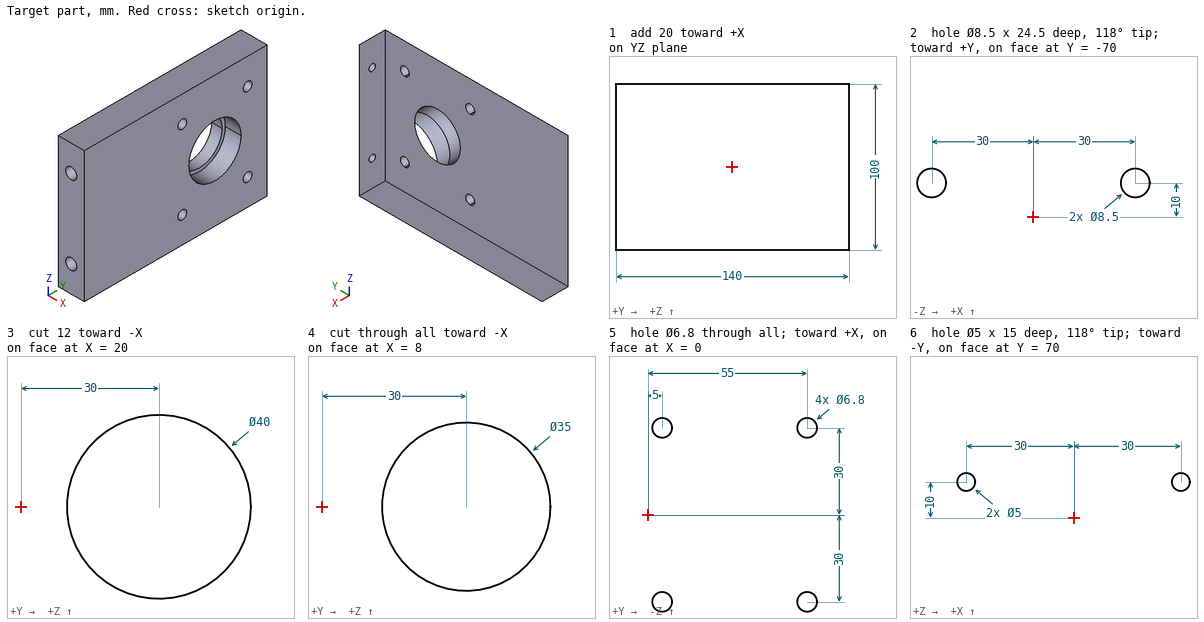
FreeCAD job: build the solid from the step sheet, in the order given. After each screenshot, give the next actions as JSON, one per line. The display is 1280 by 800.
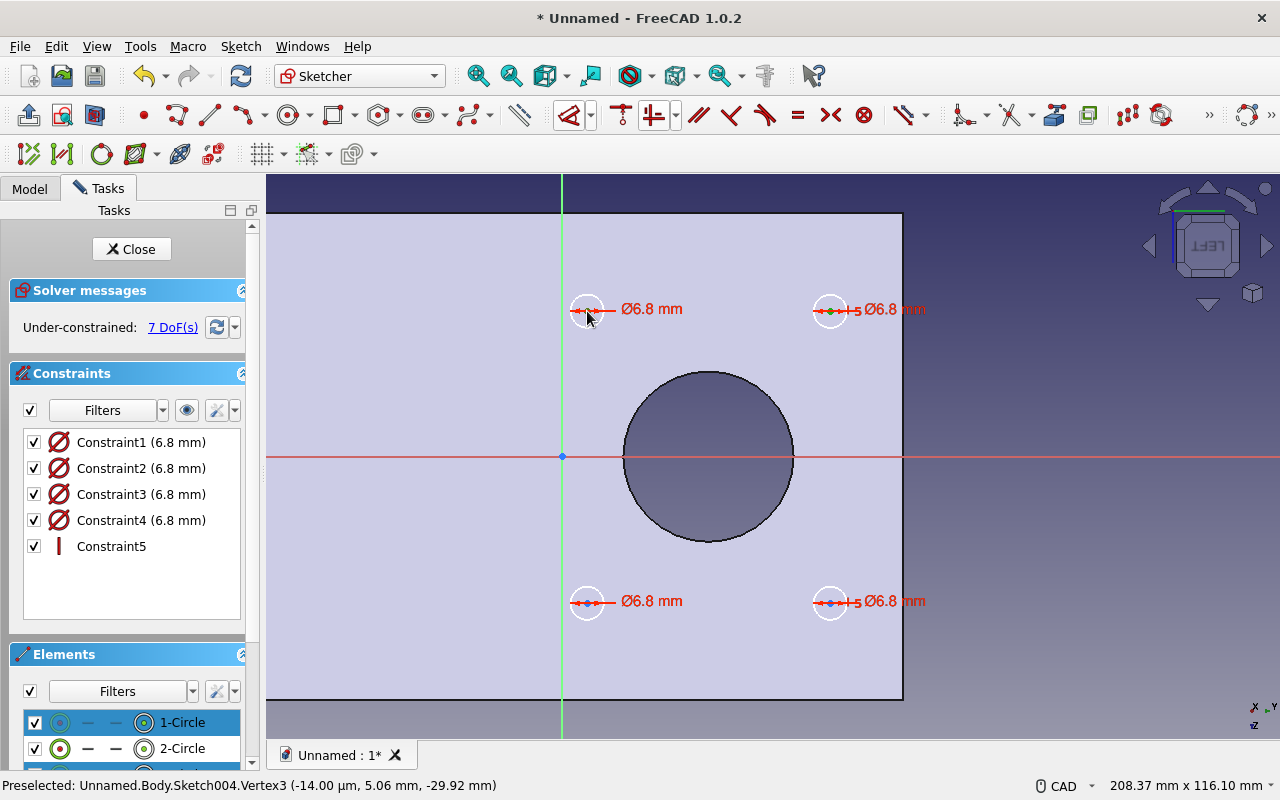
{"action": "key", "text": "h"}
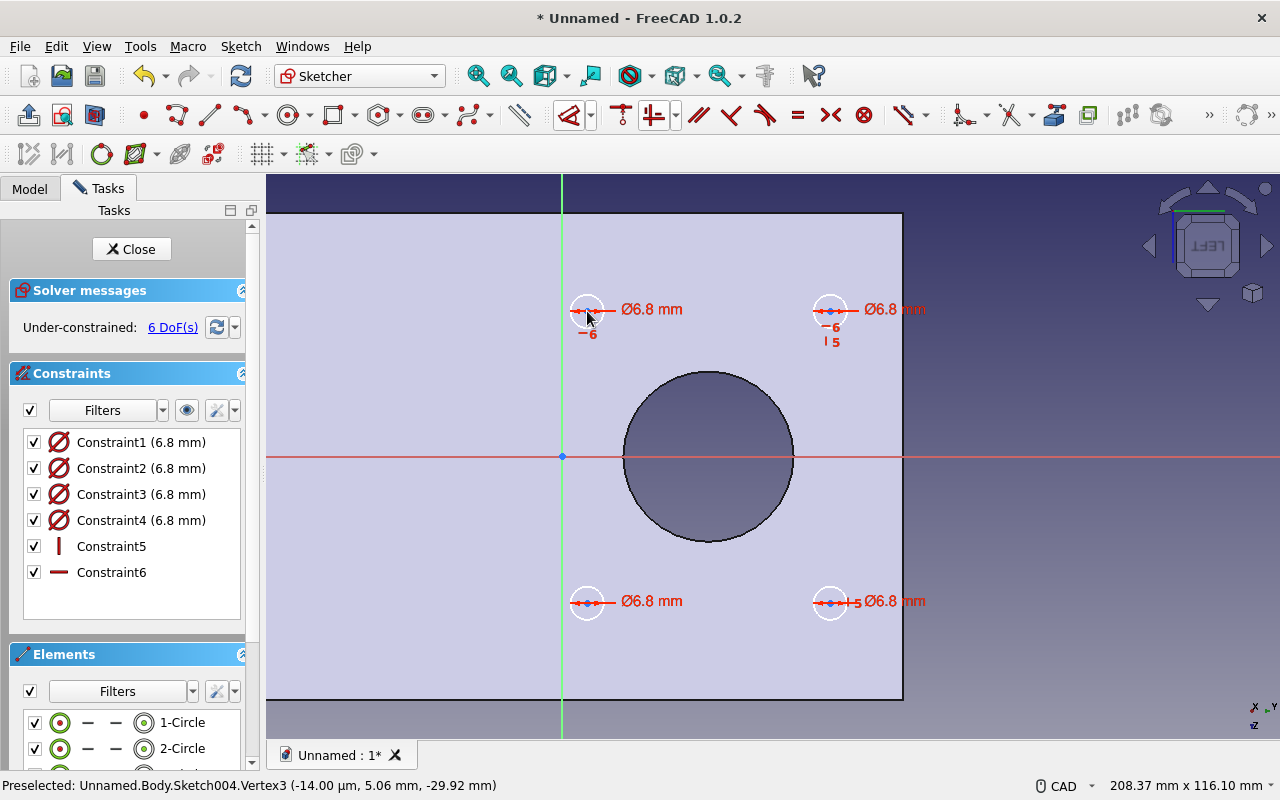
{"action": "left_click", "coordinate": [587, 311]}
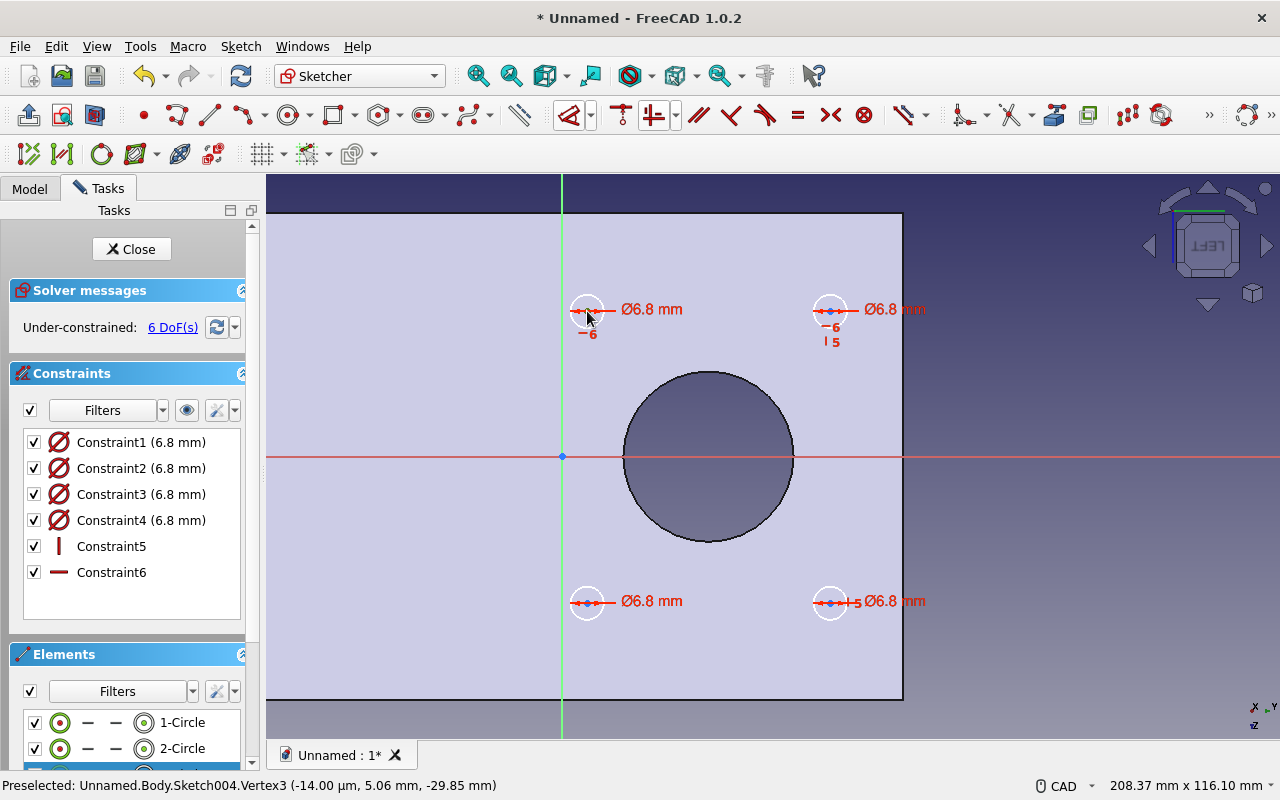
{"action": "left_click", "coordinate": [587, 603]}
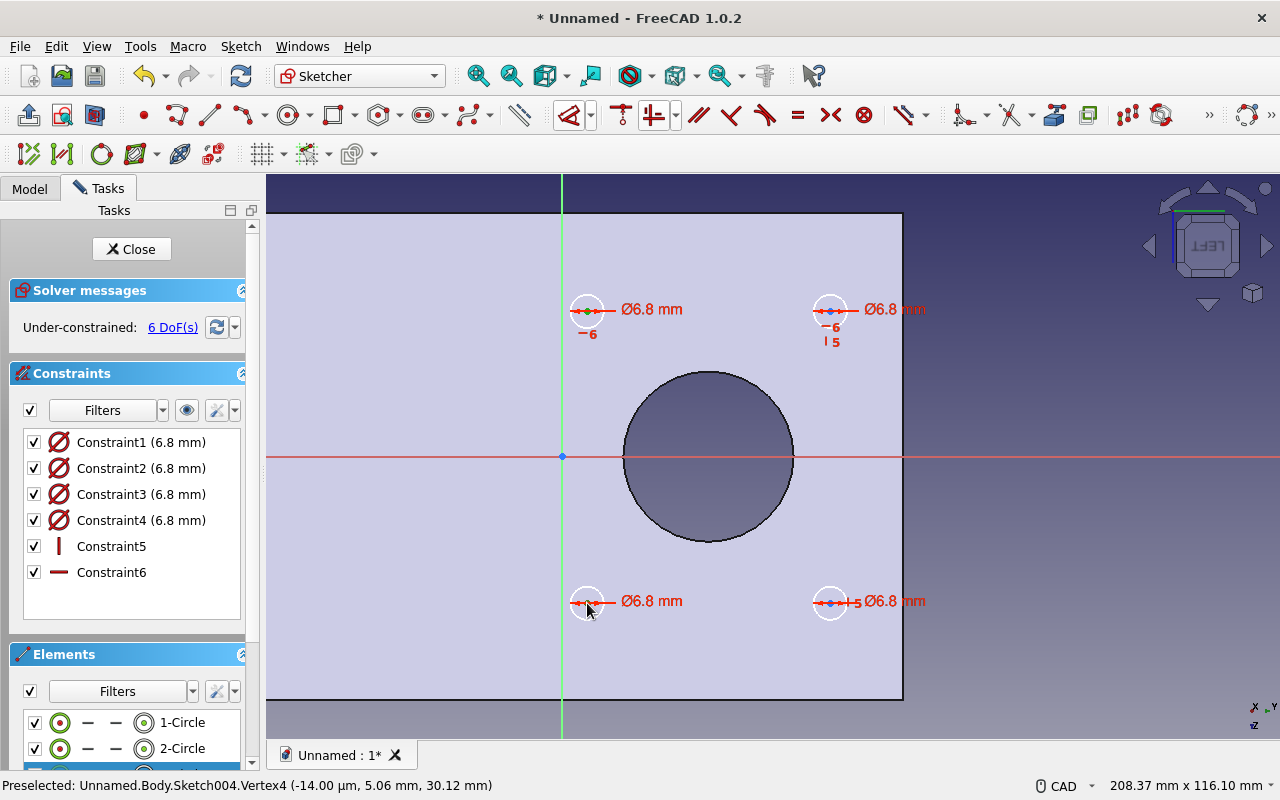
{"action": "key", "text": "v"}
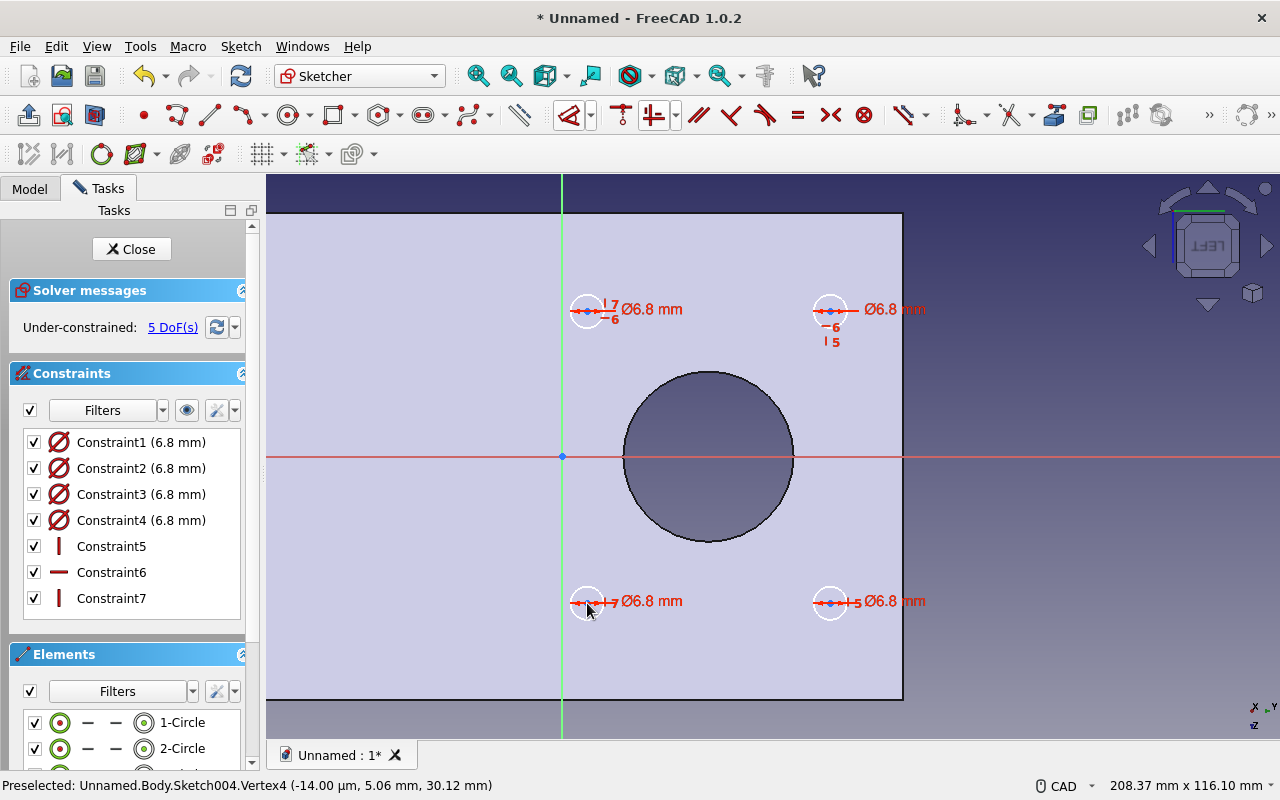
{"action": "left_click", "coordinate": [830, 603]}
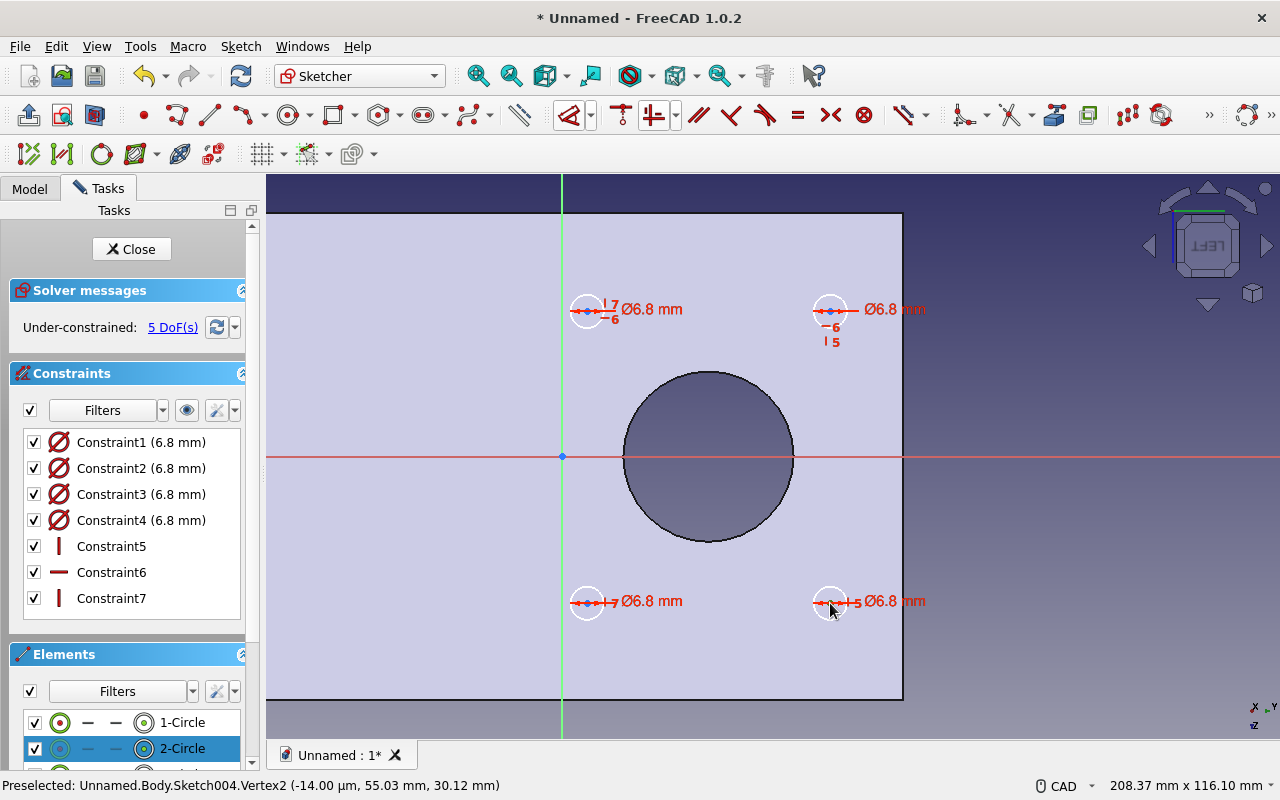
{"action": "left_click", "coordinate": [587, 603]}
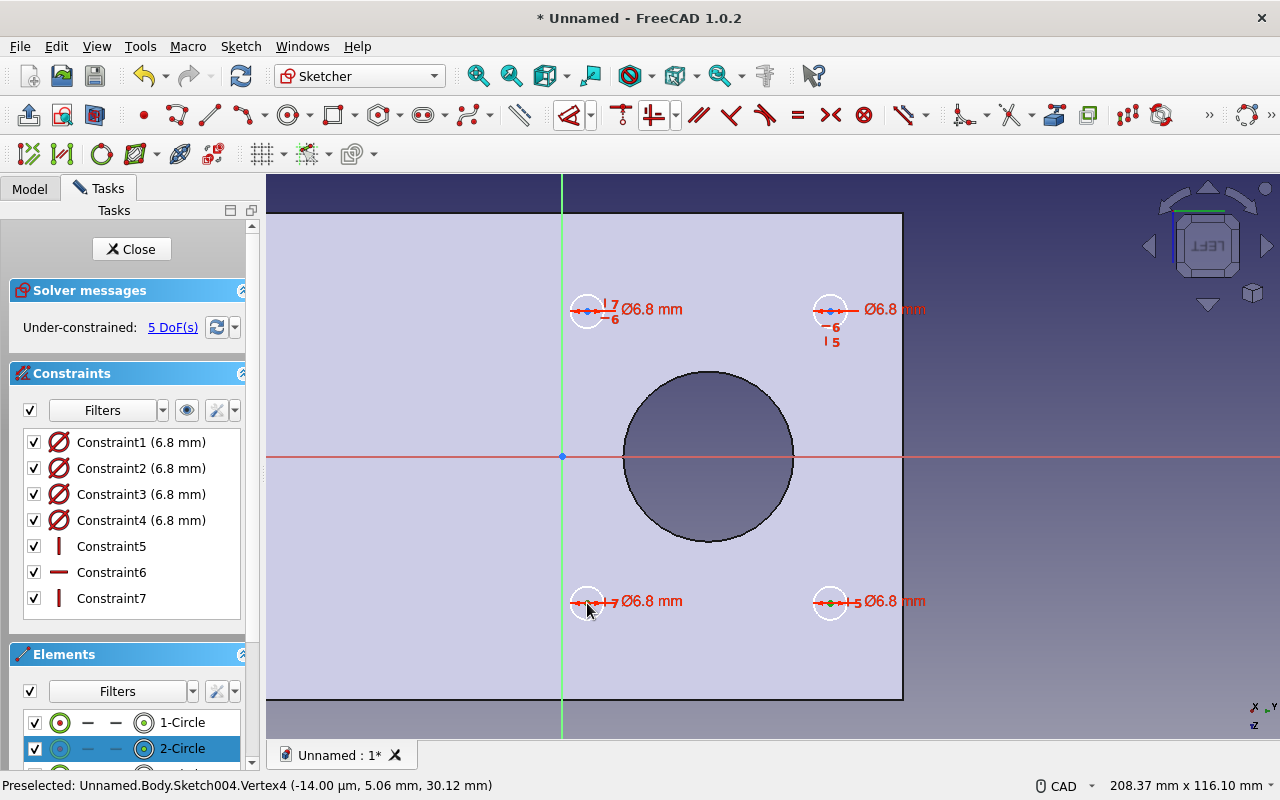
{"action": "left_click", "coordinate": [676, 116]}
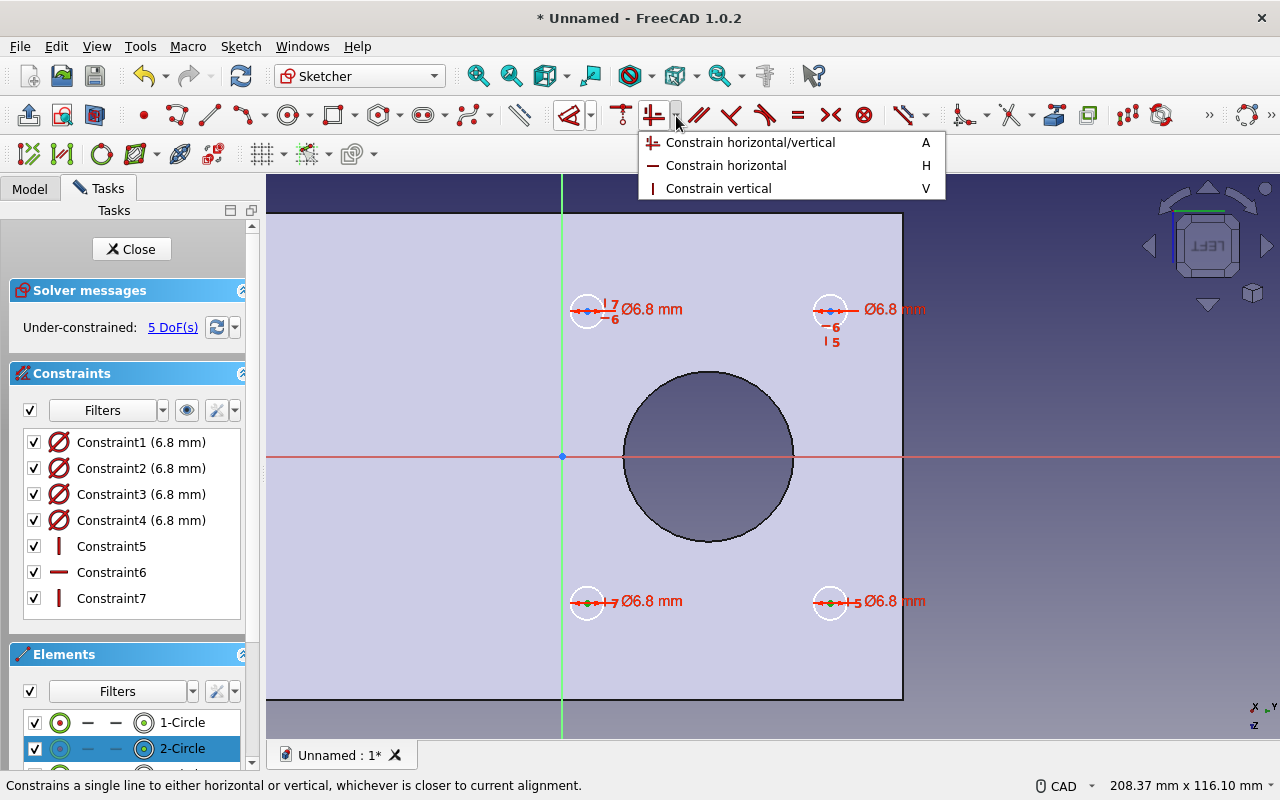
{"action": "left_click", "coordinate": [792, 166]}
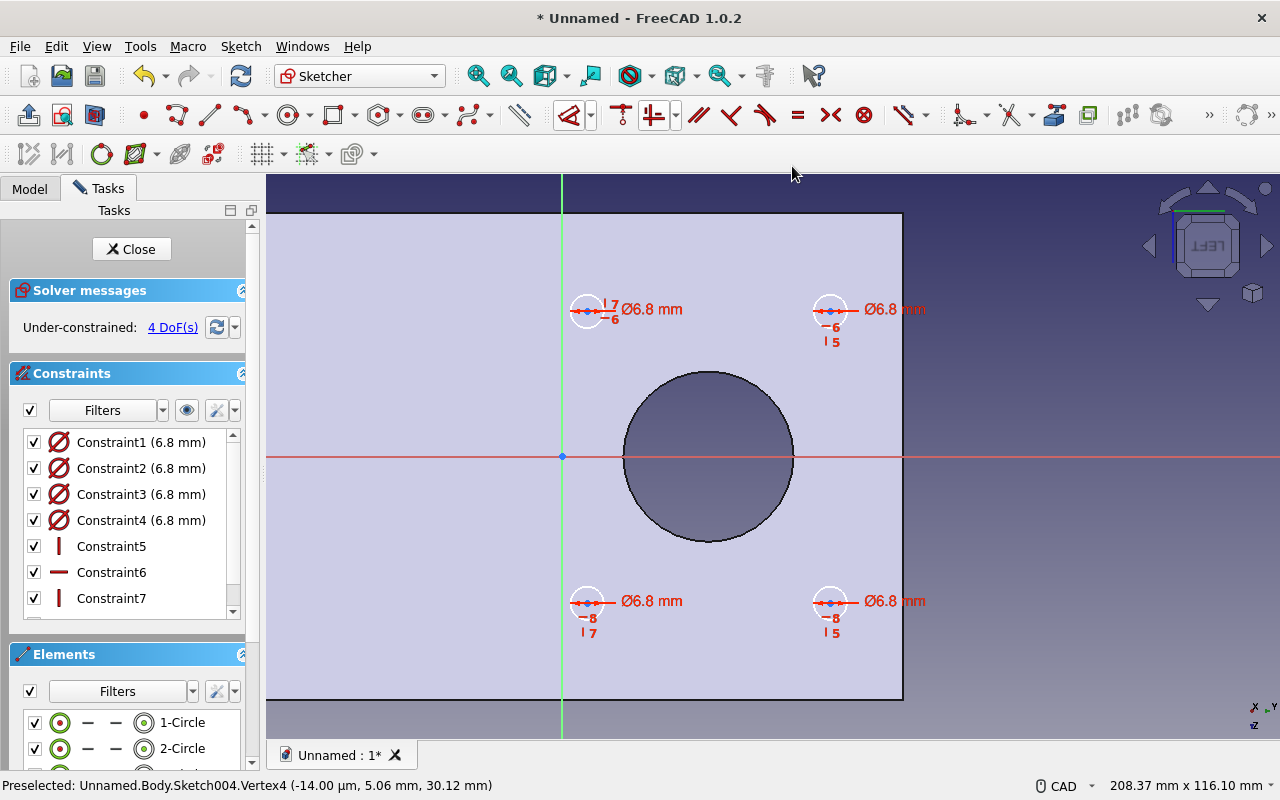
{"action": "scroll", "coordinate": [587, 311], "scroll_direction": "up", "scroll_amount": 3}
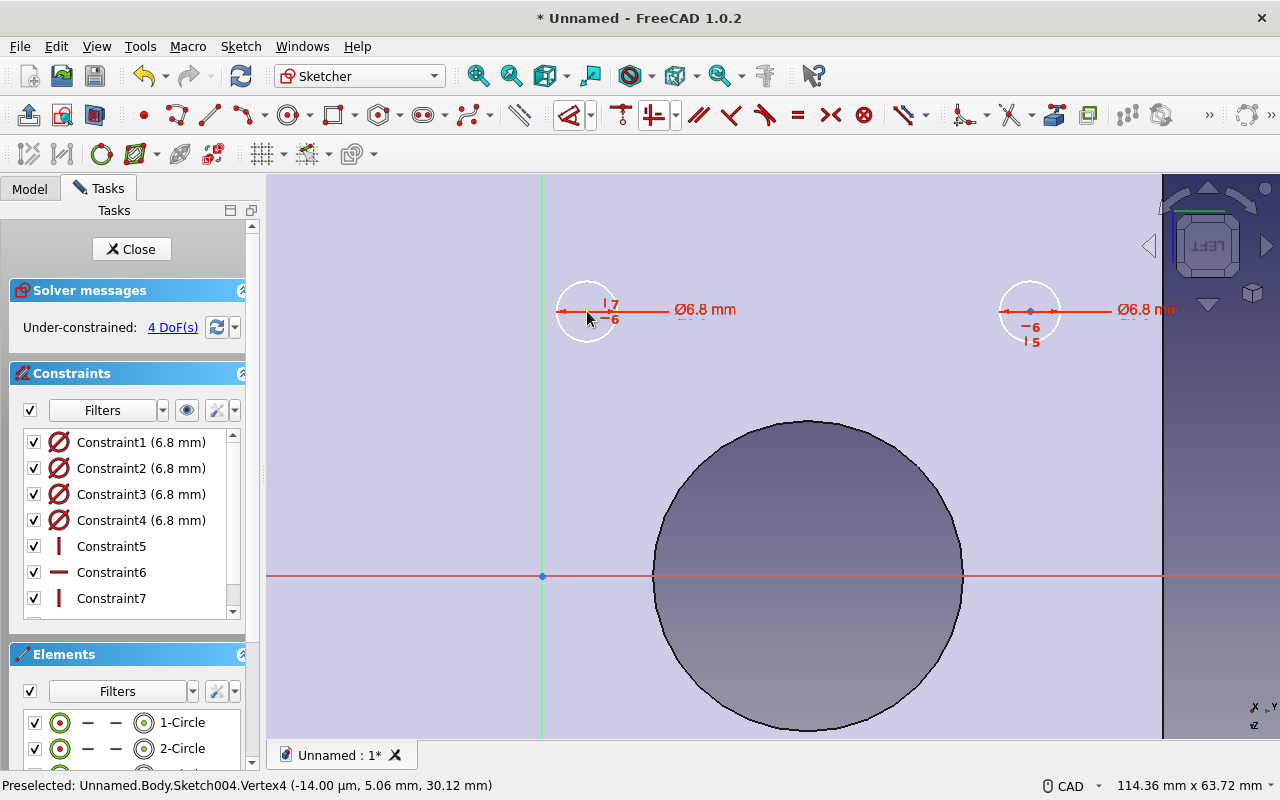
{"action": "left_click", "coordinate": [587, 312]}